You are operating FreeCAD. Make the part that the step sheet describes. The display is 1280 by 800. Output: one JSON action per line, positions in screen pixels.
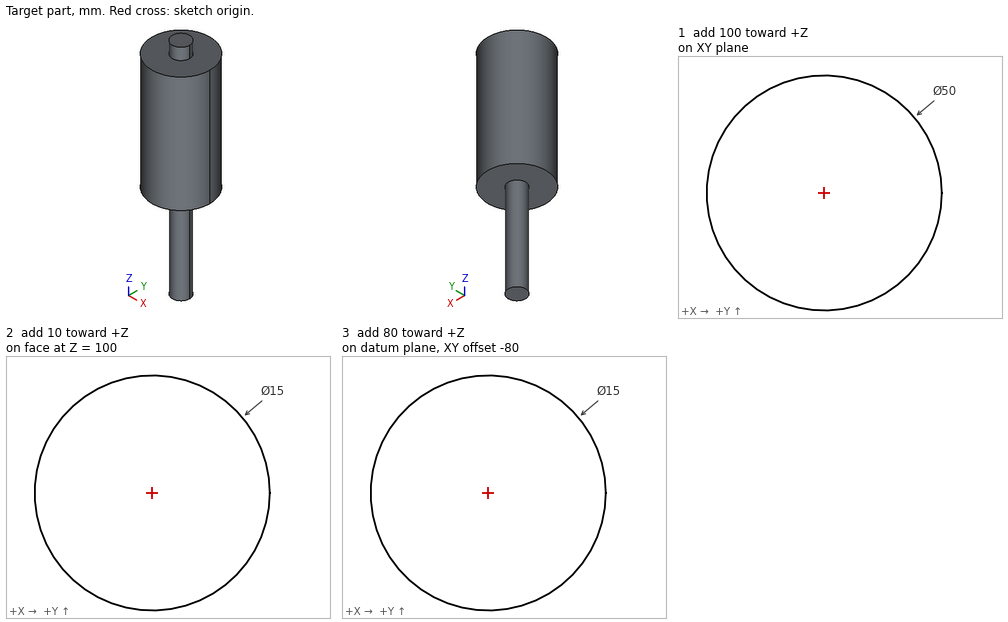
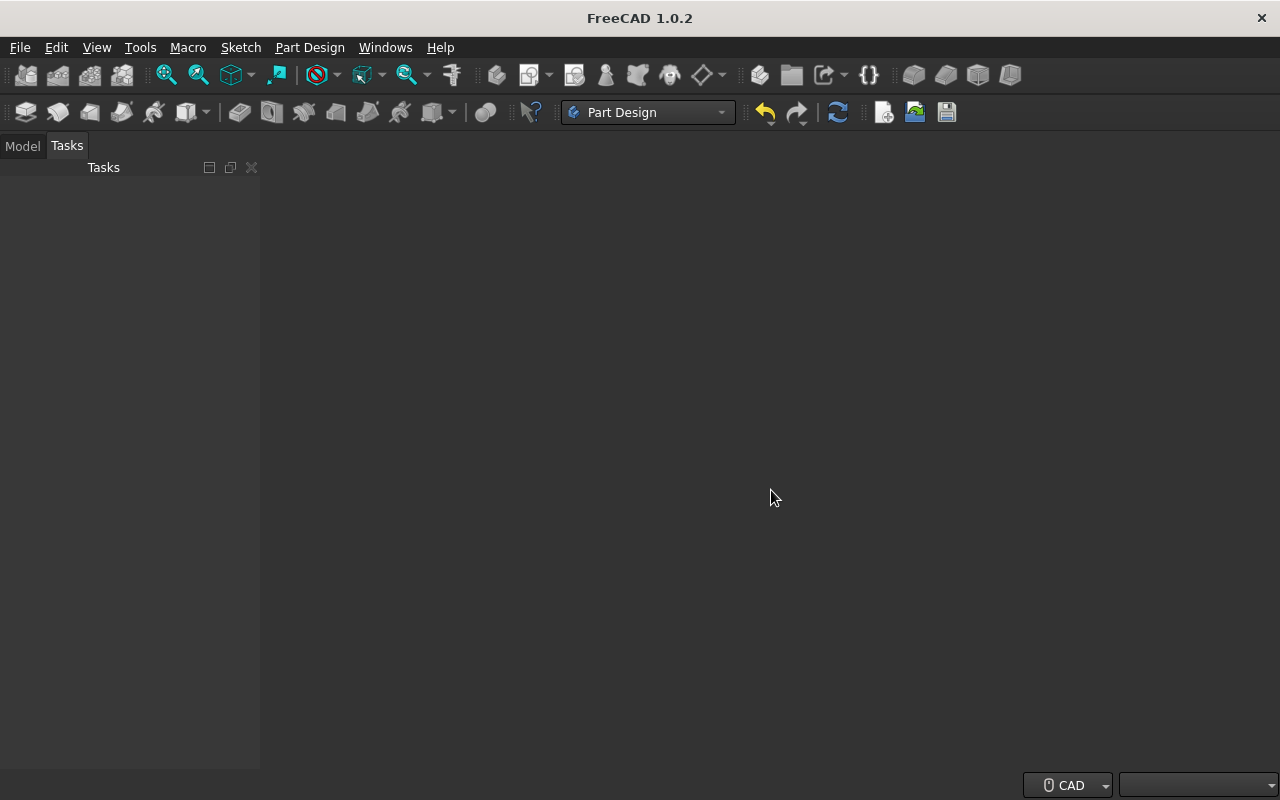
{"action": "left_click", "coordinate": [884, 112]}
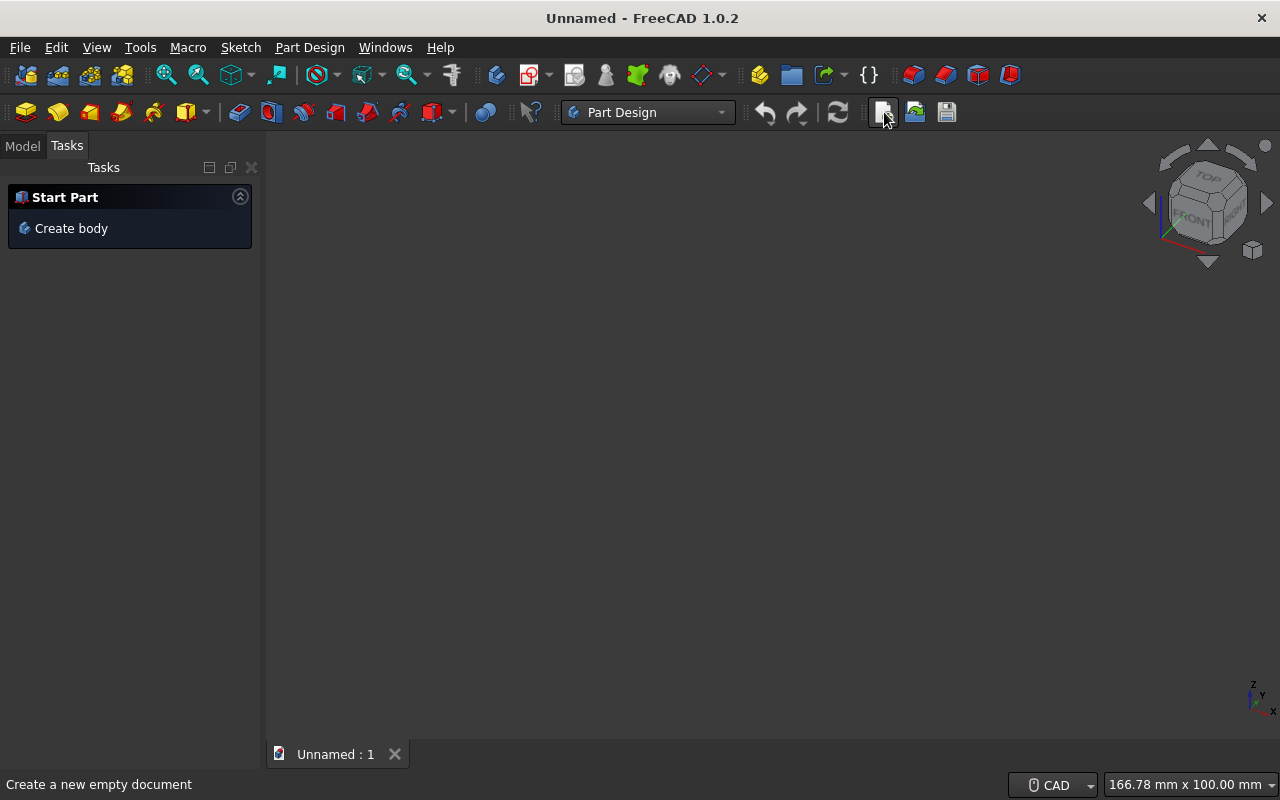
{"action": "left_click", "coordinate": [530, 76]}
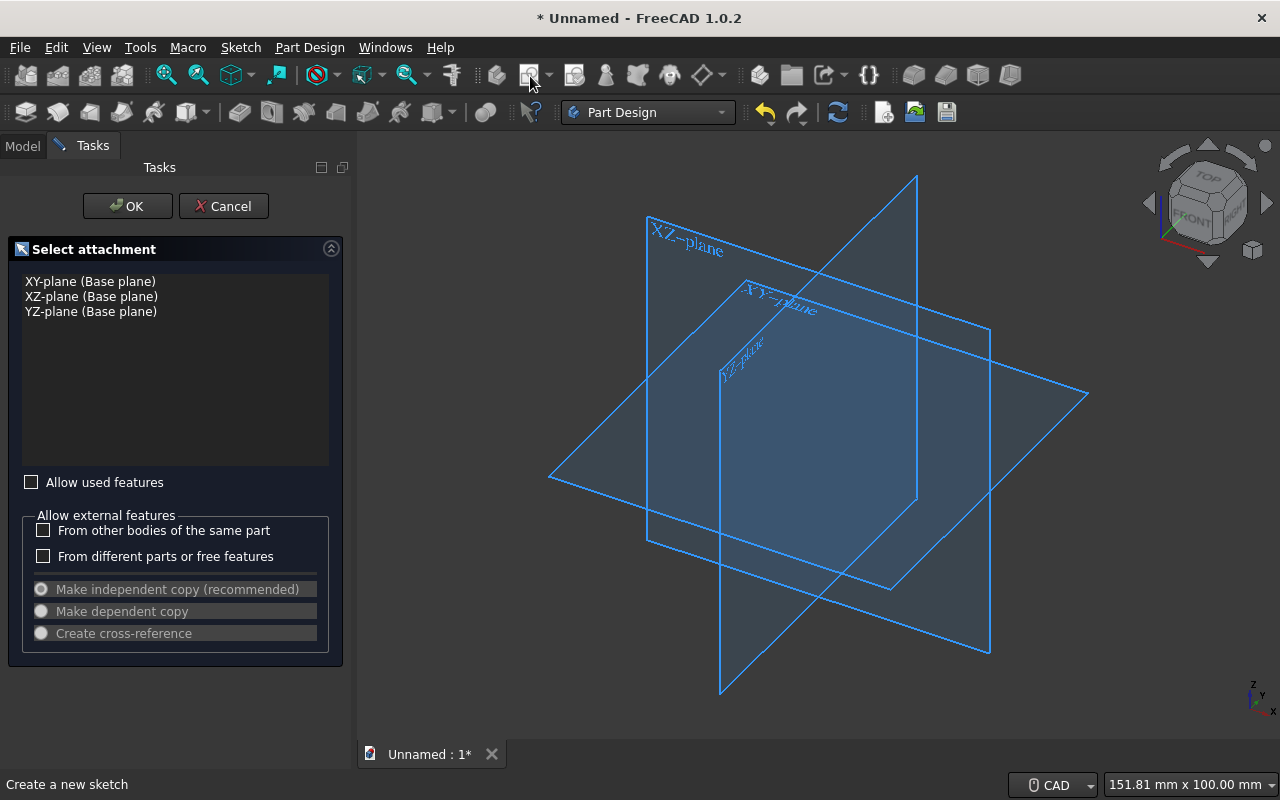
{"action": "left_click", "coordinate": [82, 282]}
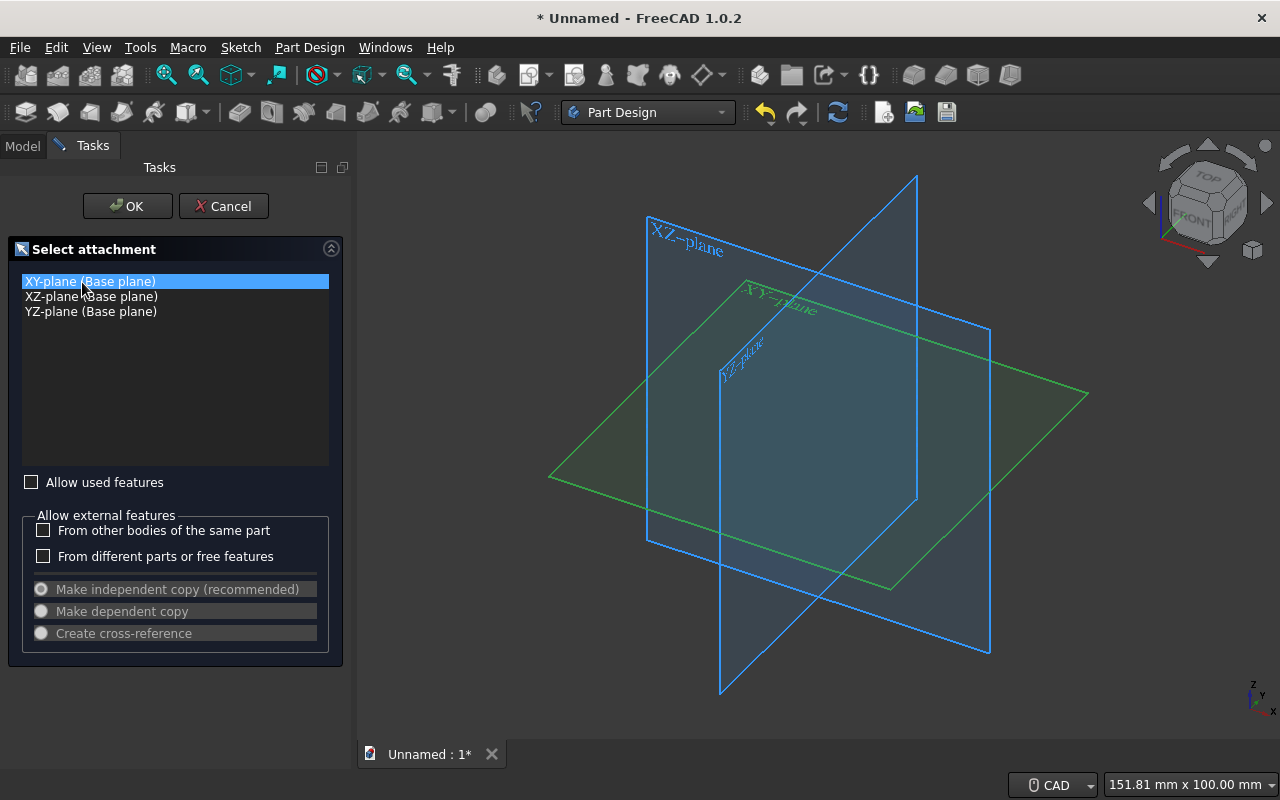
{"action": "left_click", "coordinate": [128, 206]}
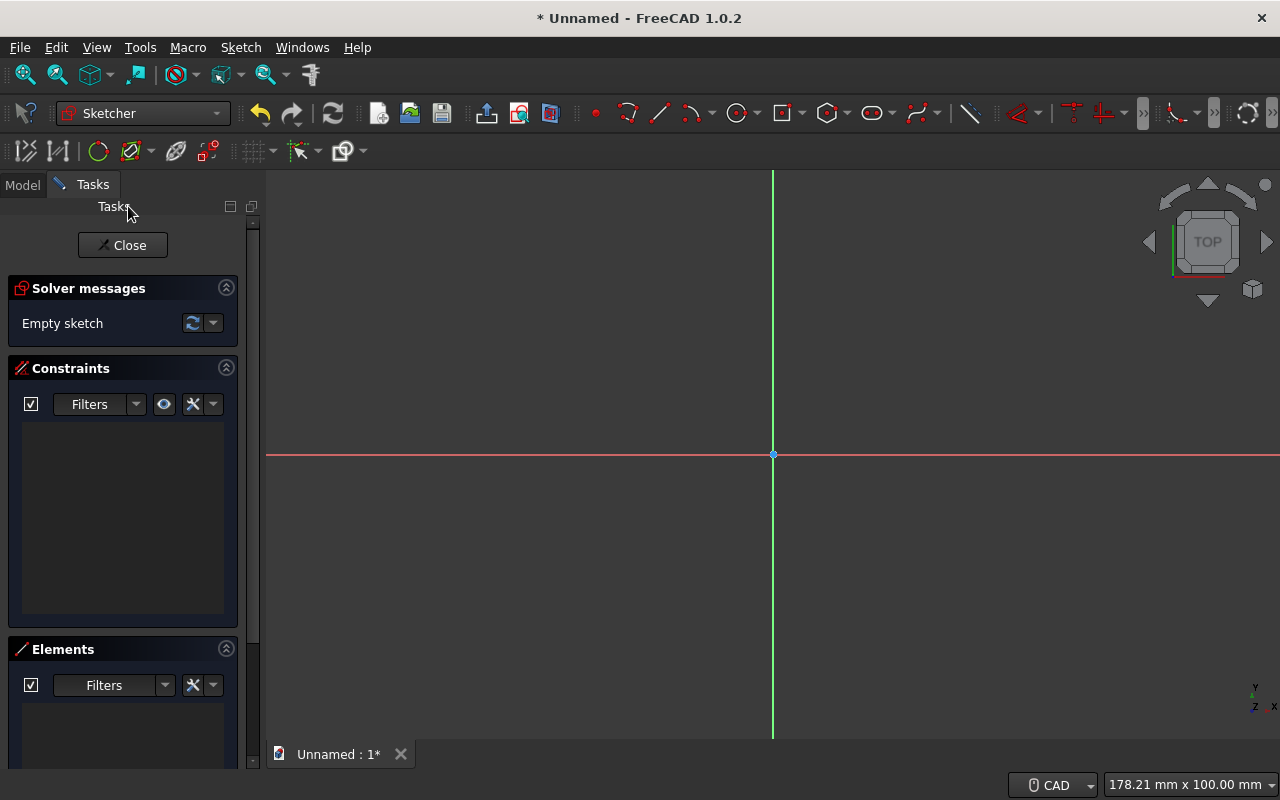
{"action": "key", "text": "g c"}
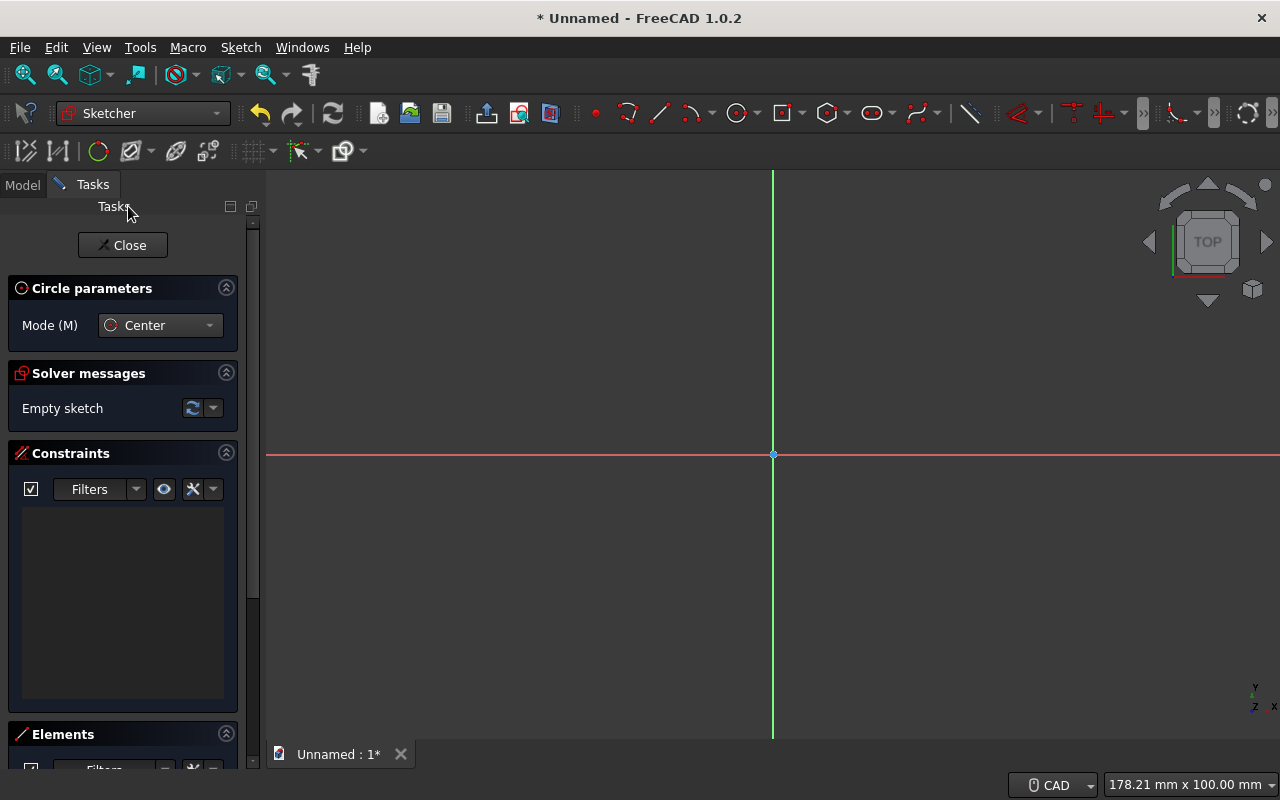
{"action": "left_click", "coordinate": [773, 454]}
{"action": "mouse_move", "coordinate": [874, 354]}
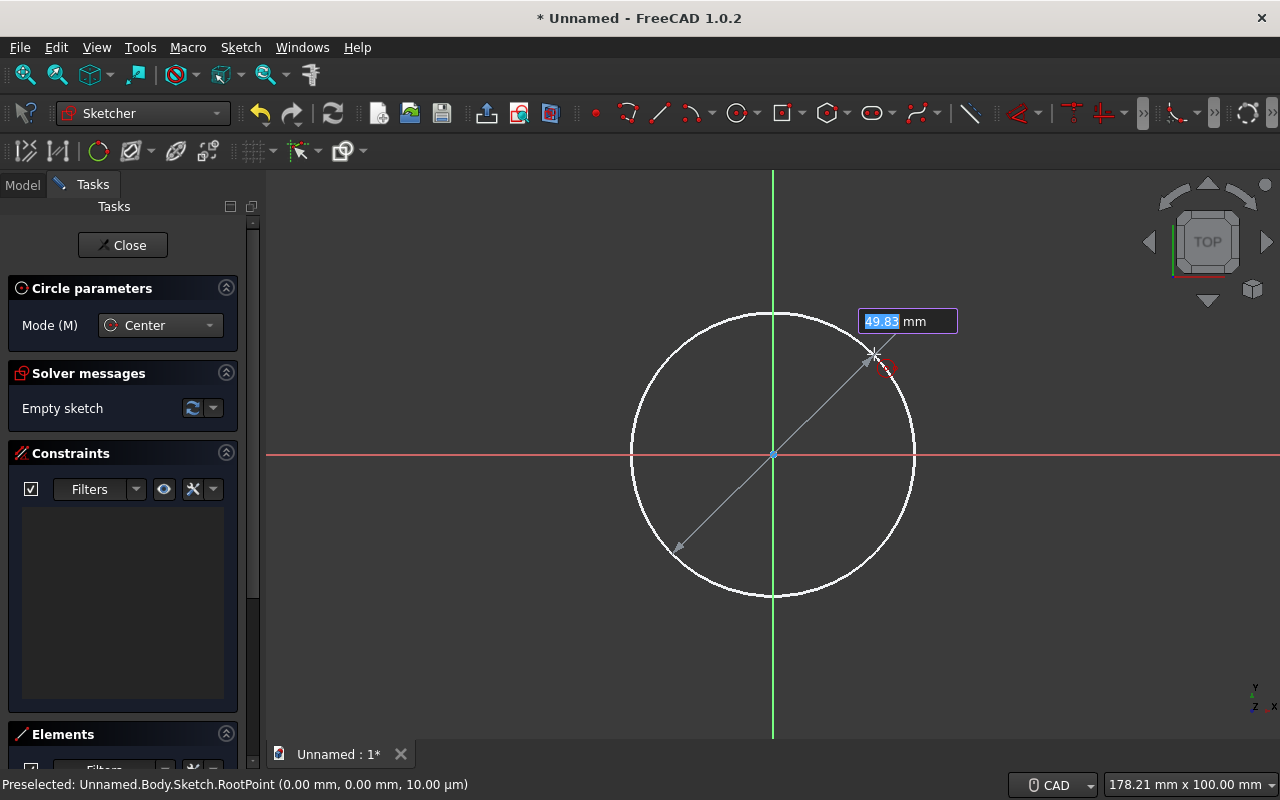
{"action": "type", "text": "50"}
{"action": "key", "text": "Return"}
{"action": "key", "text": "Escape"}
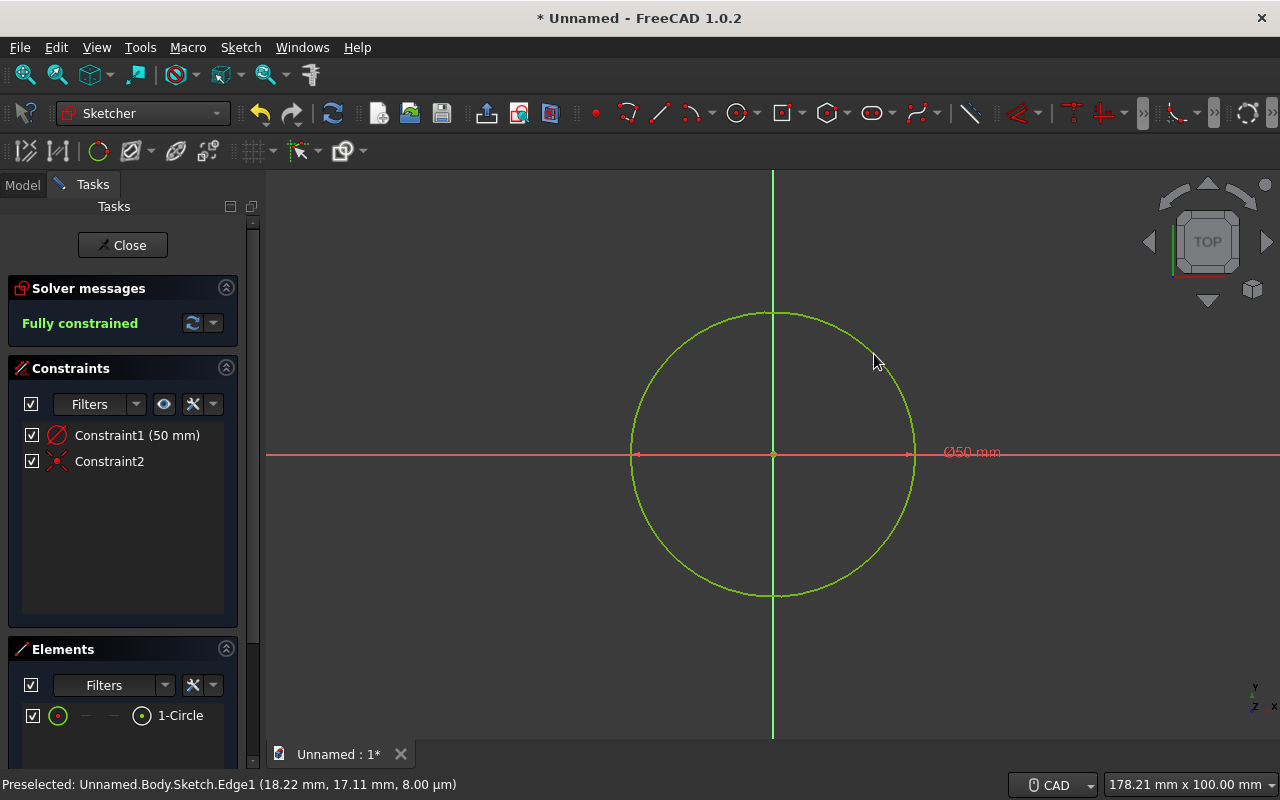
{"action": "left_click", "coordinate": [123, 245]}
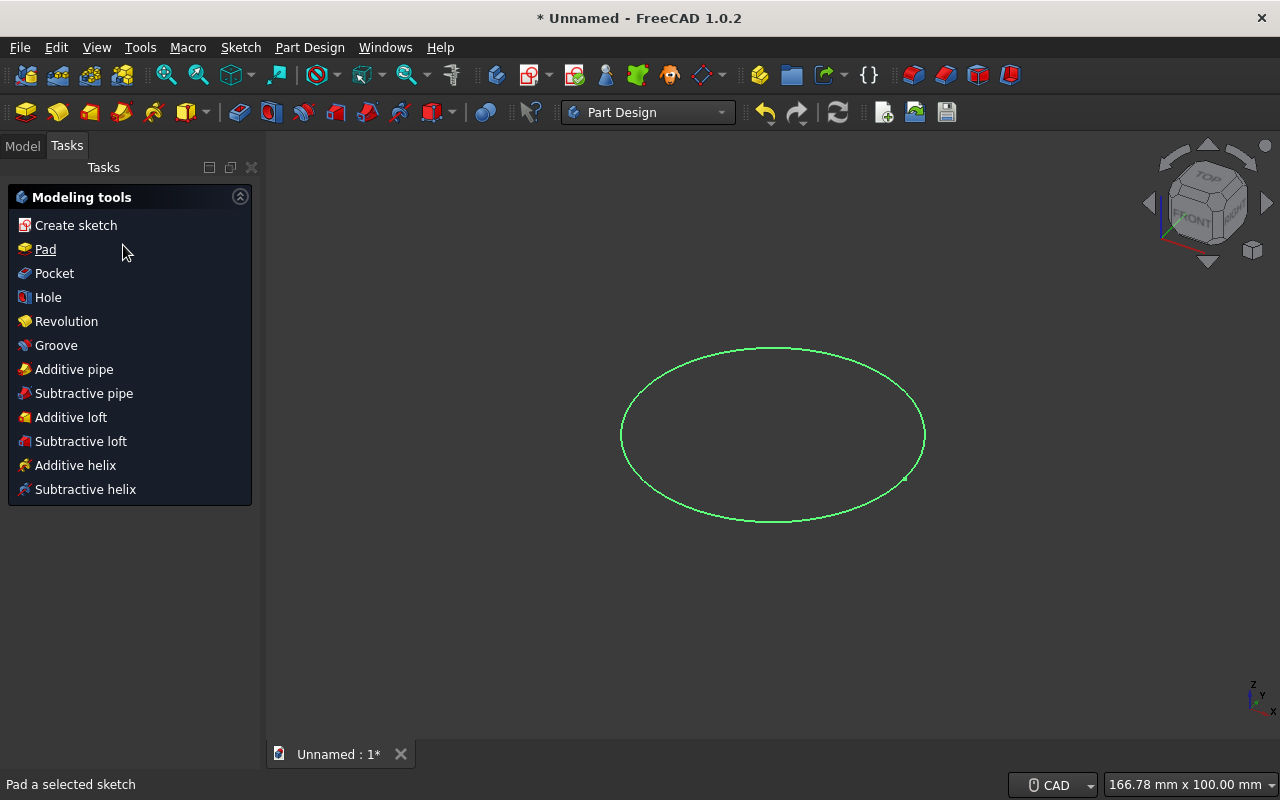
{"action": "left_click", "coordinate": [26, 112]}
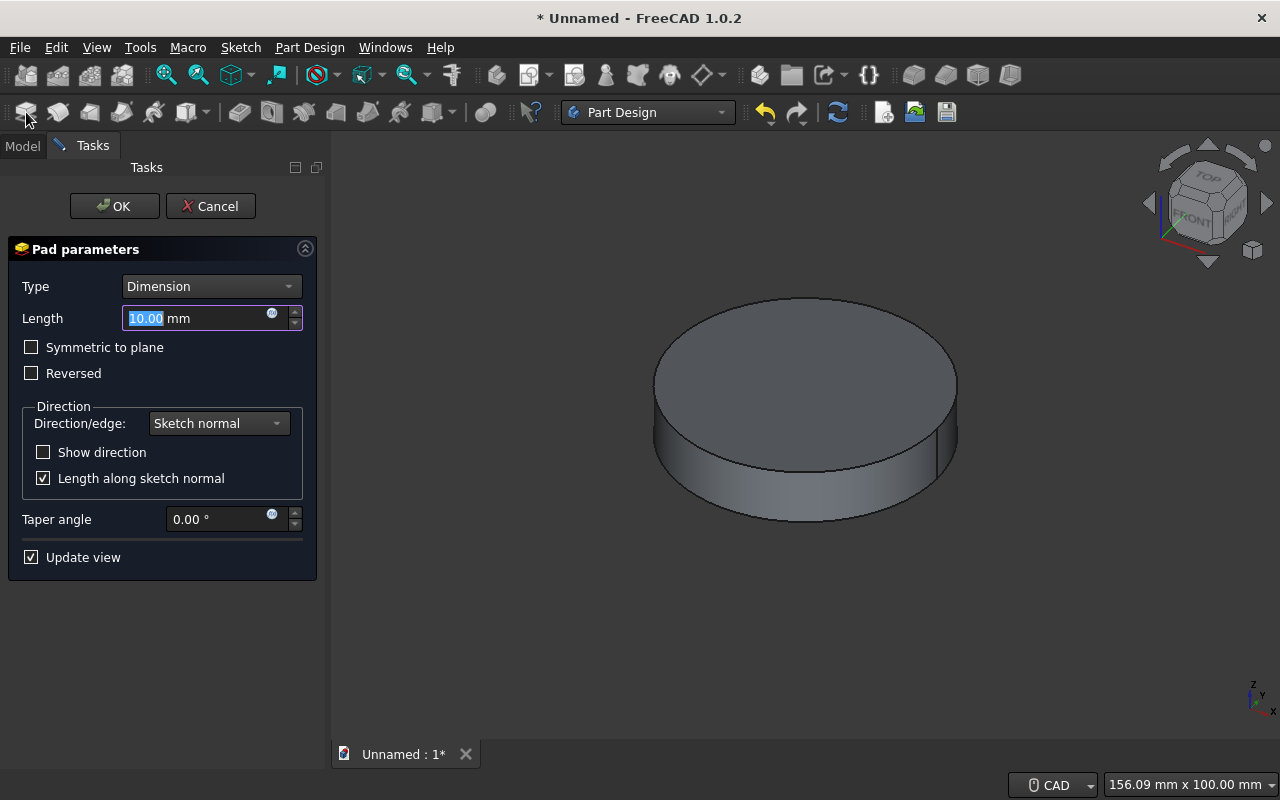
{"action": "type", "text": "100"}
{"action": "key", "text": "Tab"}